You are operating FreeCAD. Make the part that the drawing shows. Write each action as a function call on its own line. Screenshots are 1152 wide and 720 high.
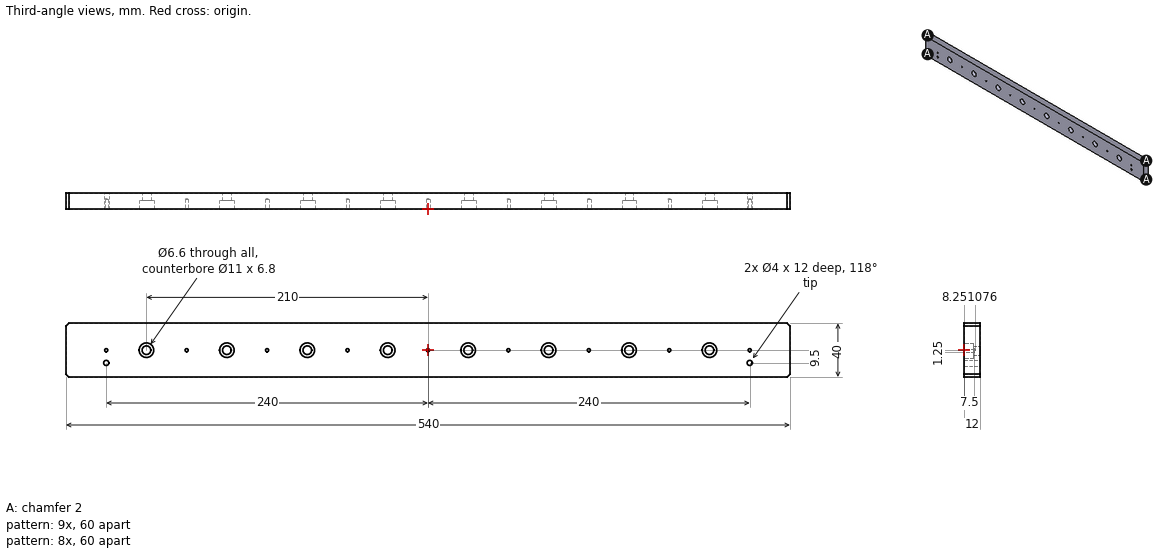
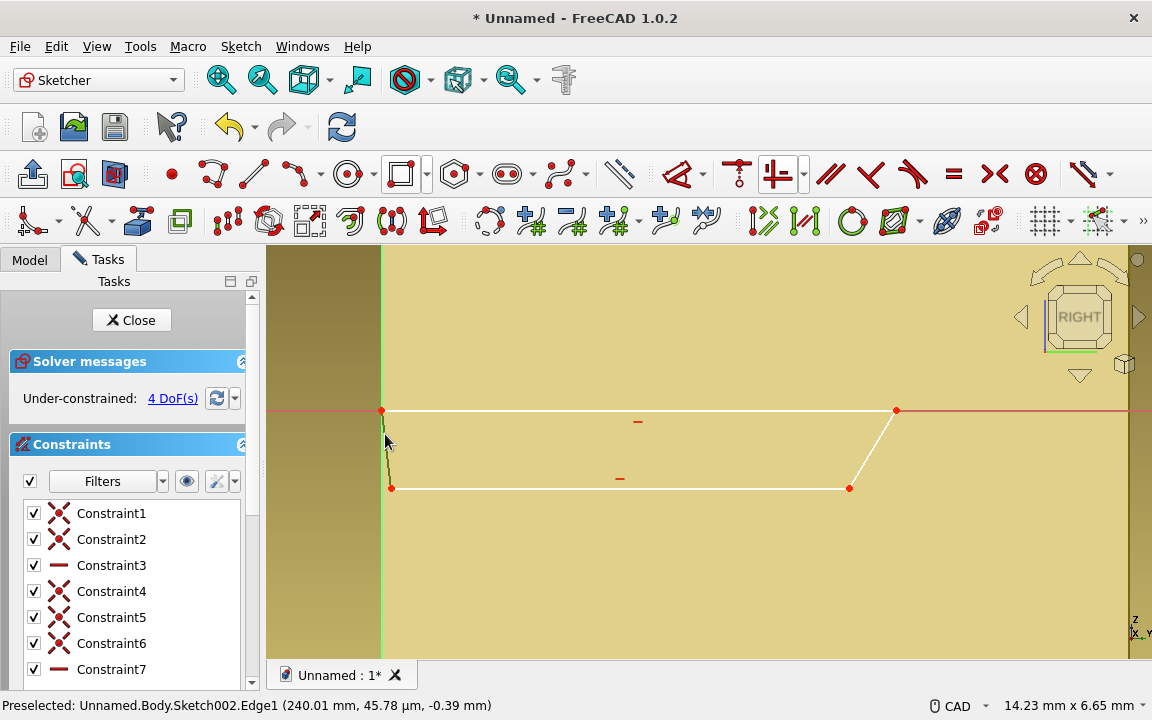
click(804, 174)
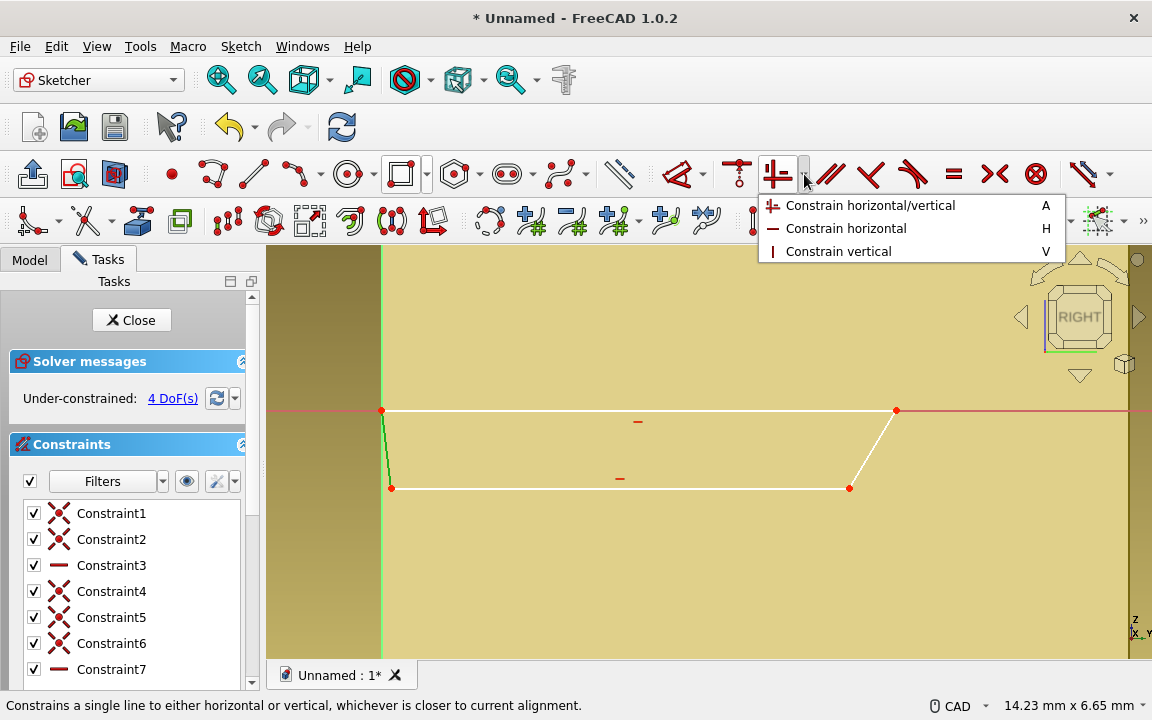
click(912, 252)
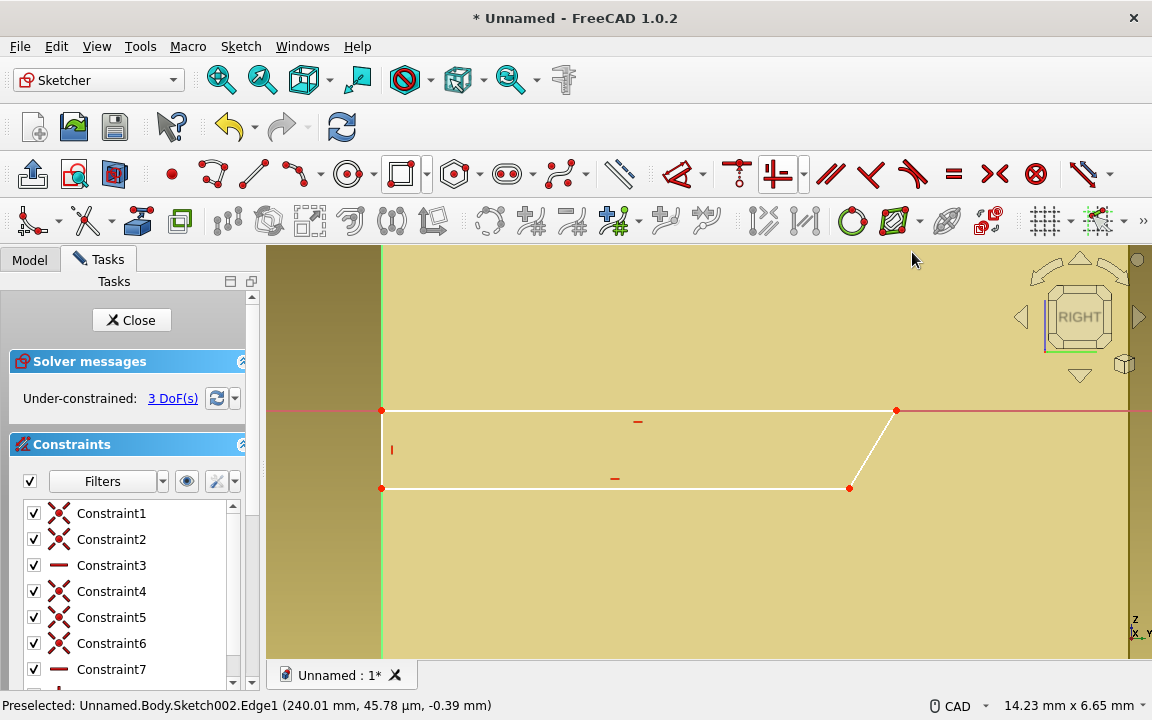
click(676, 174)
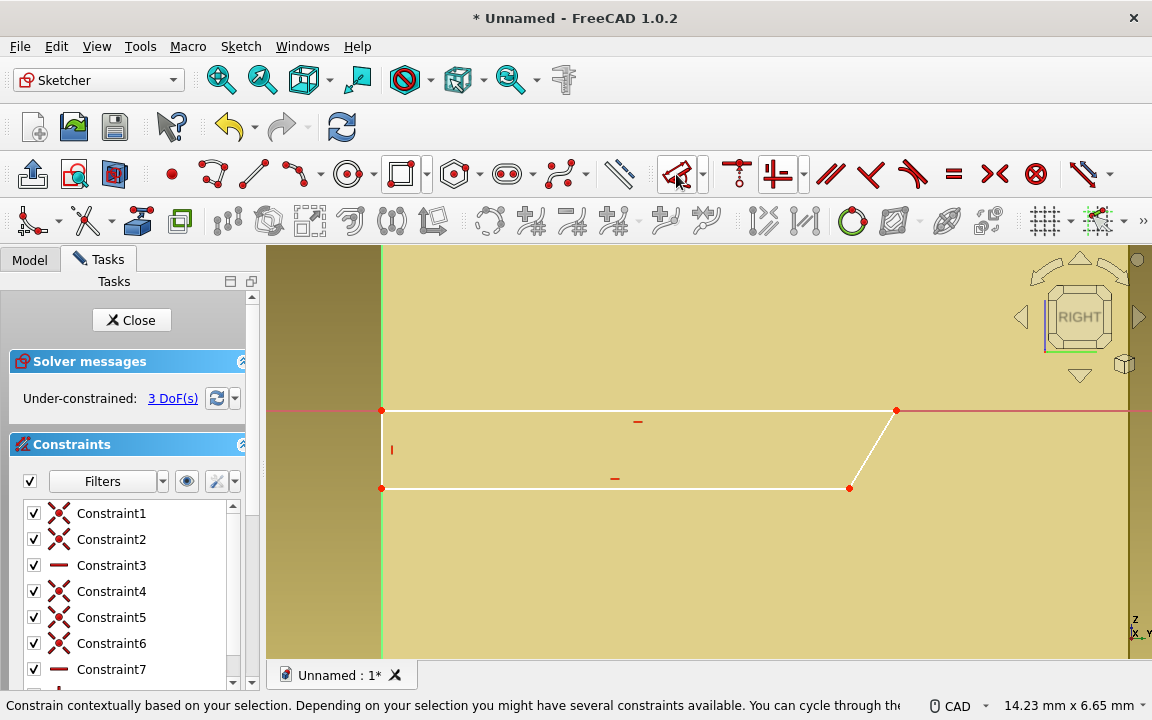
click(522, 489)
click(615, 523)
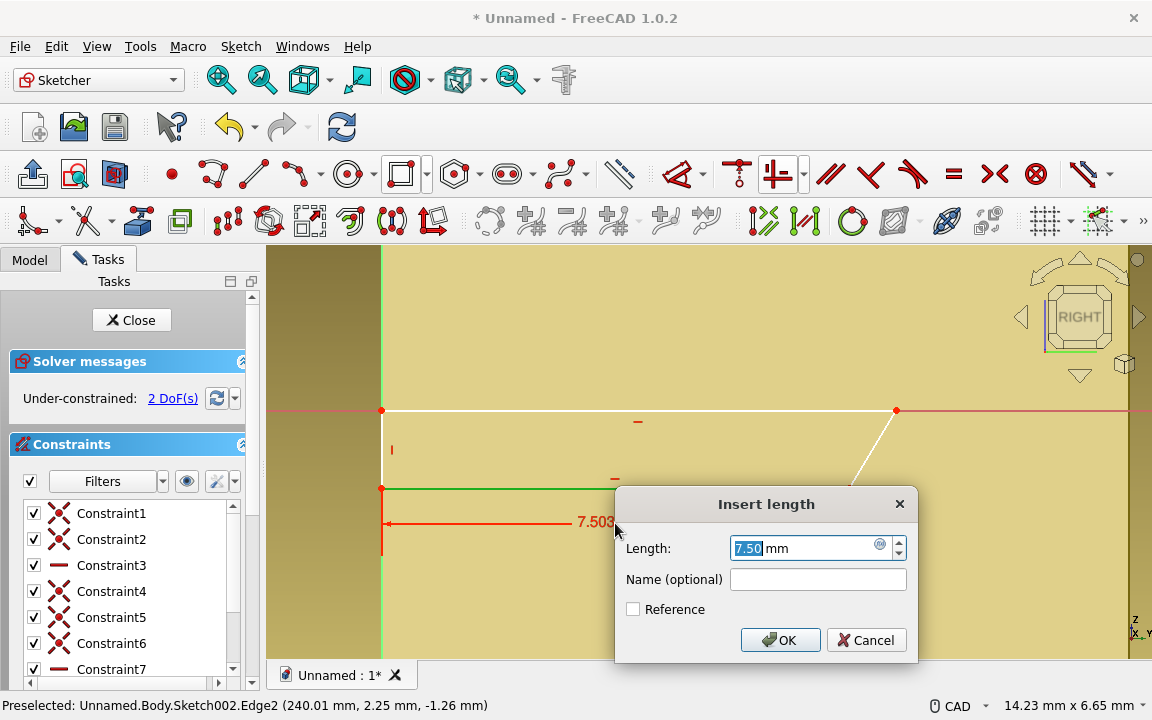
text(7.5)
key(Return)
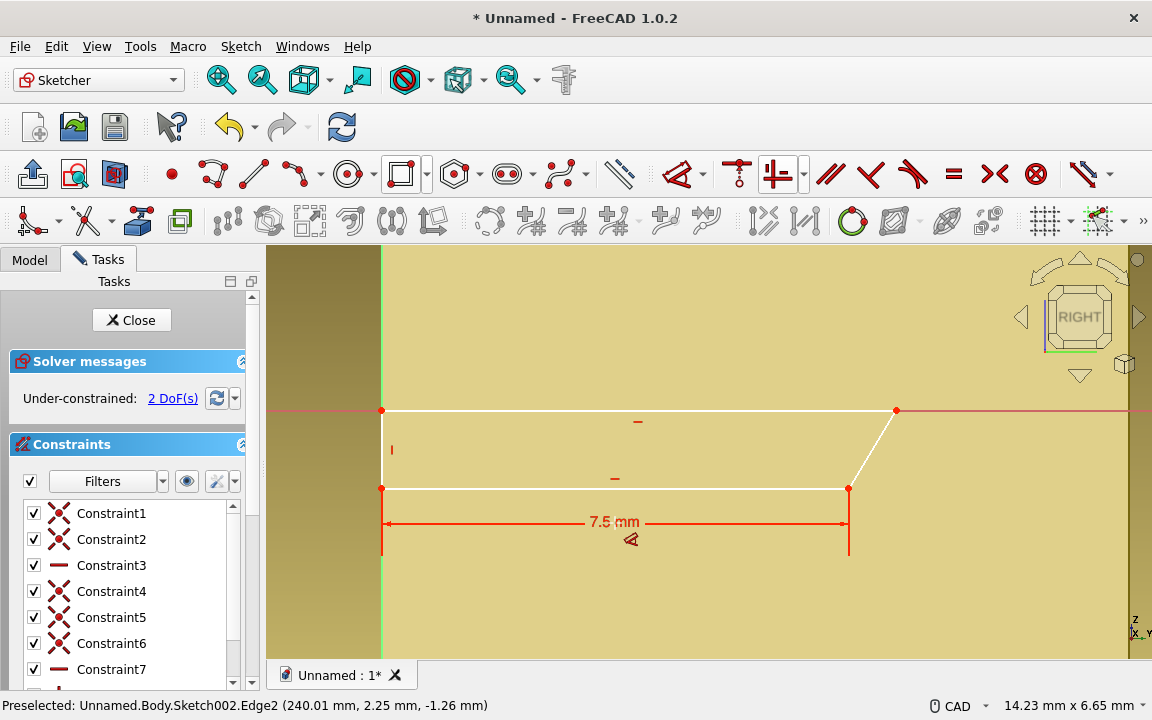
click(382, 434)
click(348, 450)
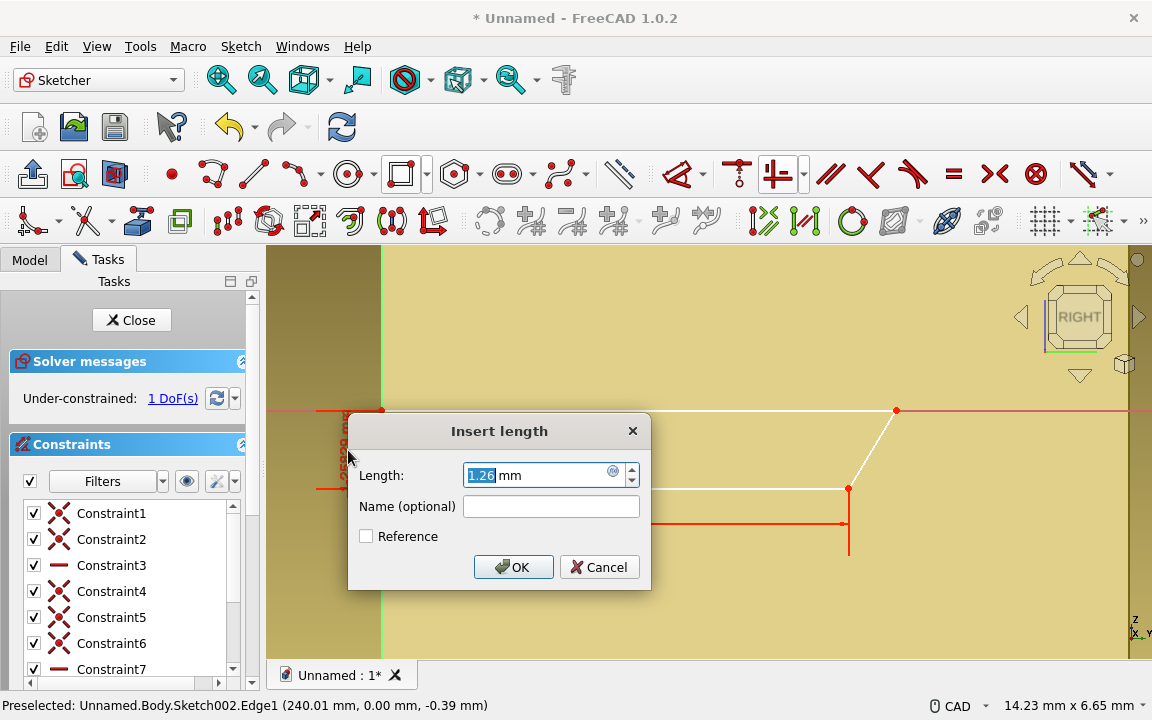
text(1.25)
key(Return)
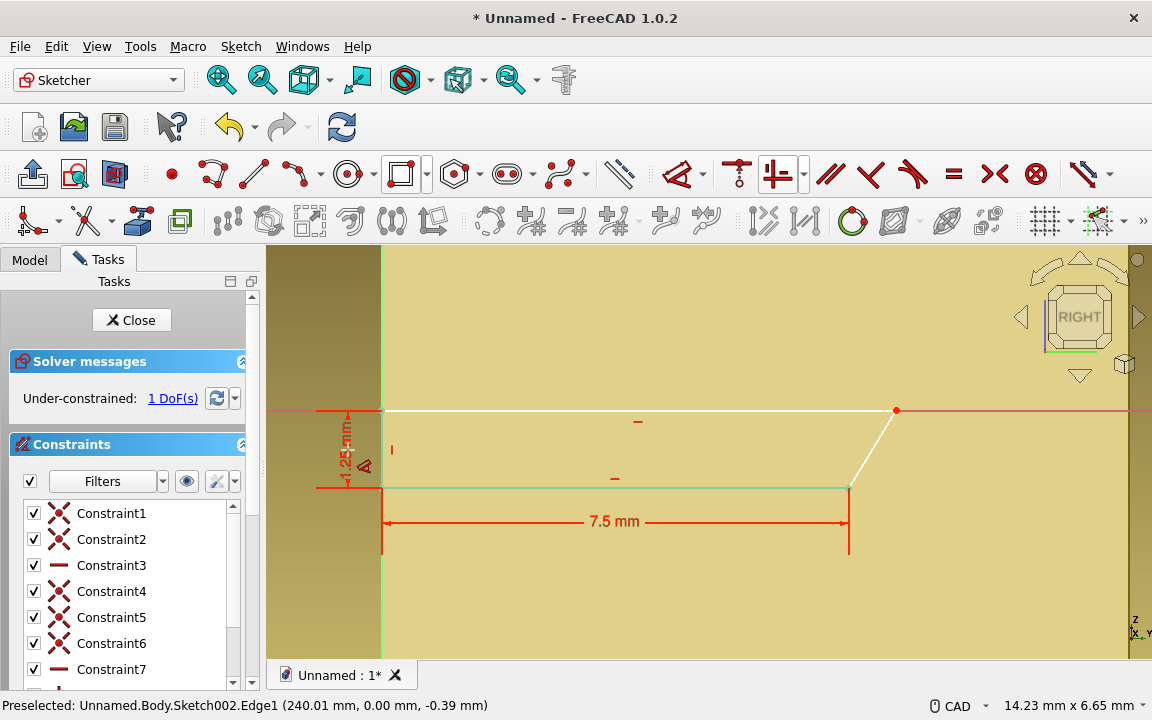
click(742, 411)
click(639, 377)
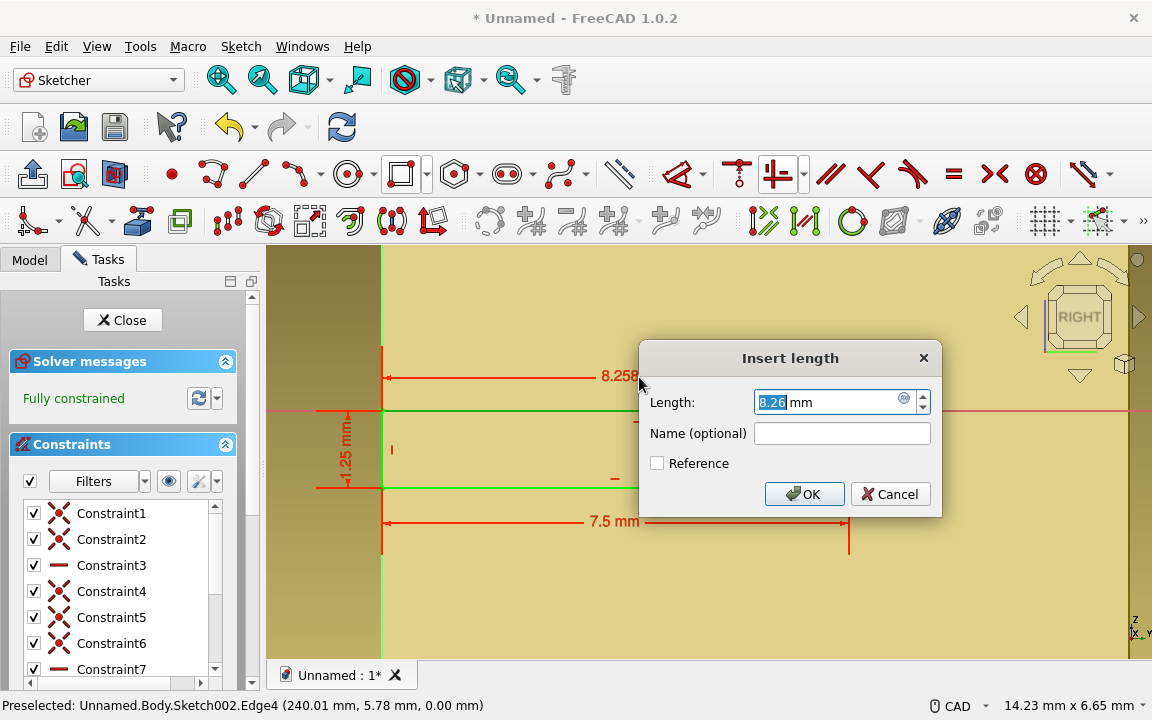
text(8.251076)
key(Return)
key(Escape)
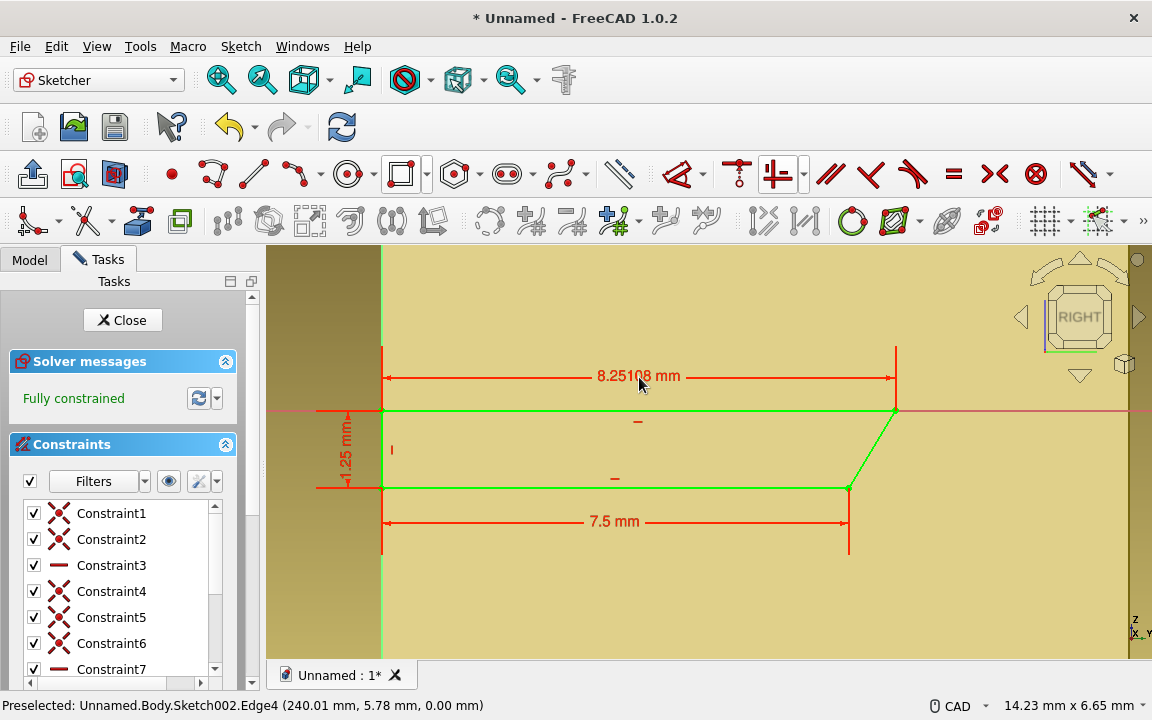
click(123, 320)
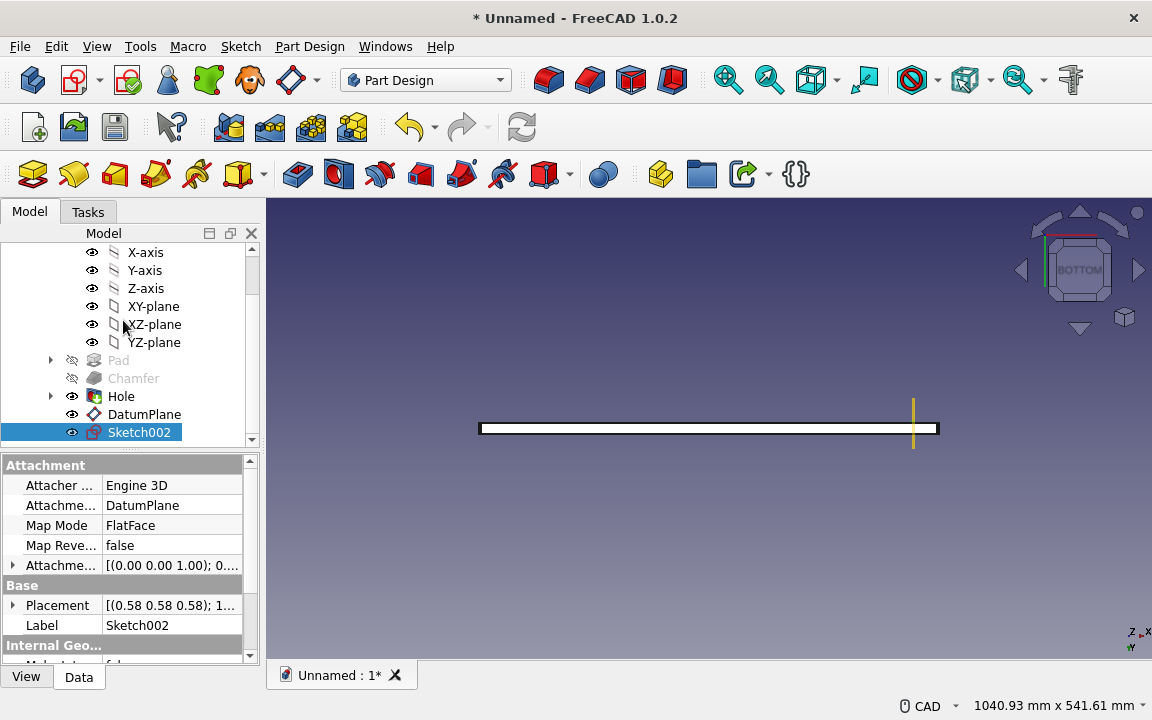
click(380, 174)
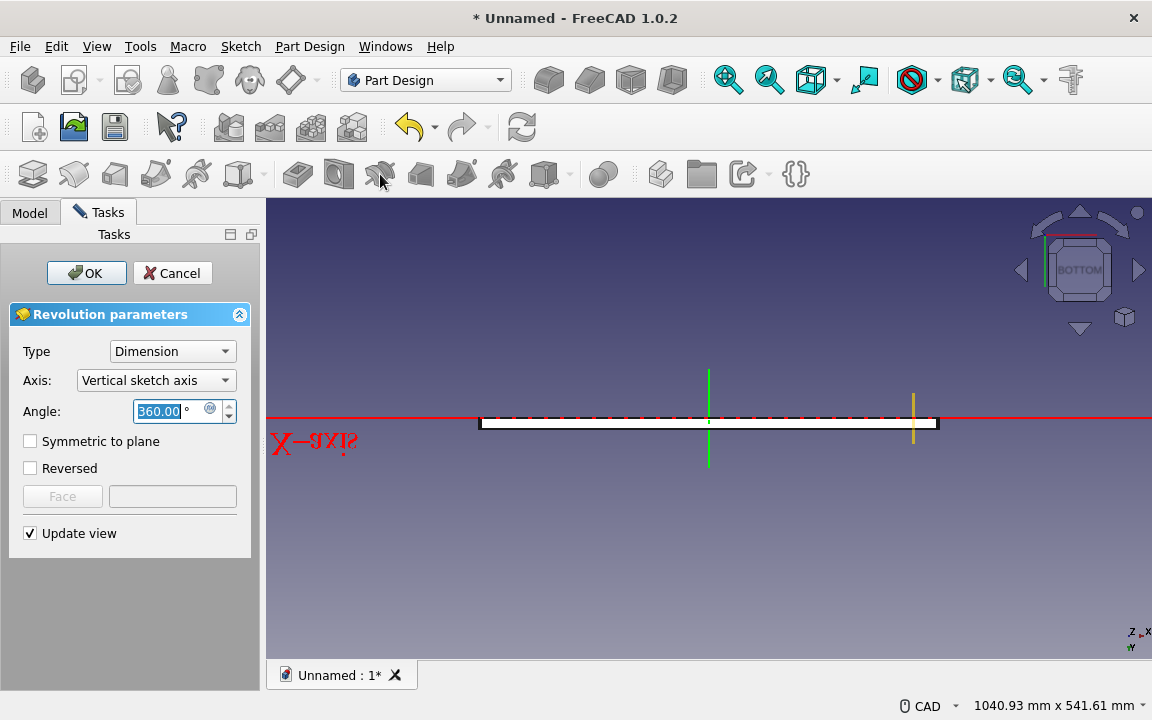
click(157, 380)